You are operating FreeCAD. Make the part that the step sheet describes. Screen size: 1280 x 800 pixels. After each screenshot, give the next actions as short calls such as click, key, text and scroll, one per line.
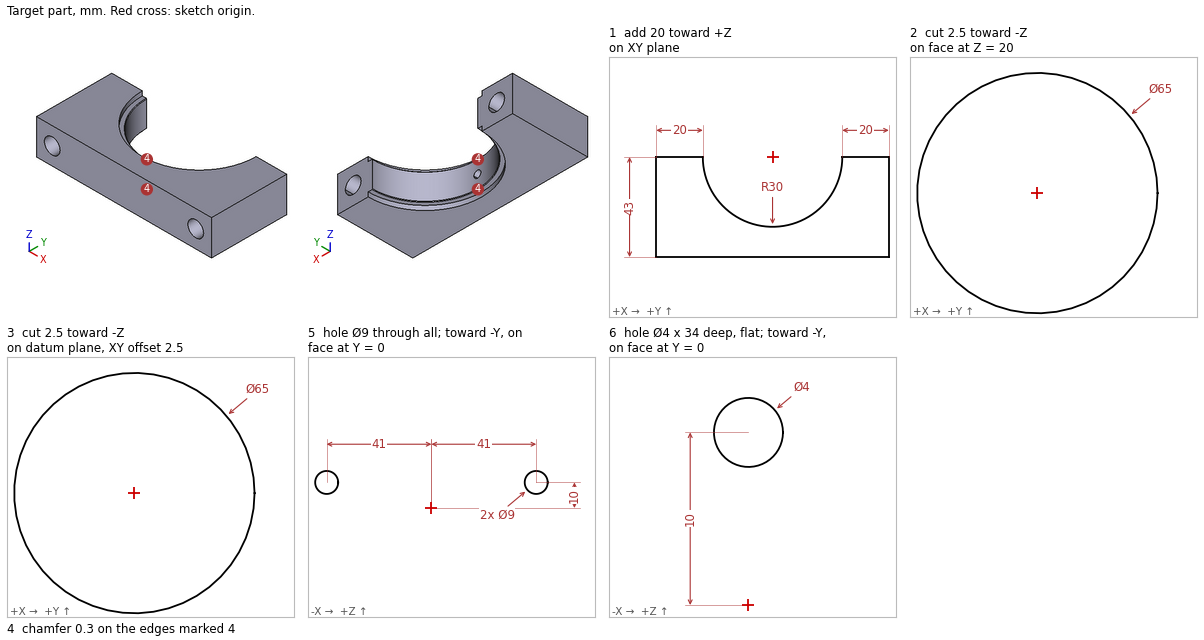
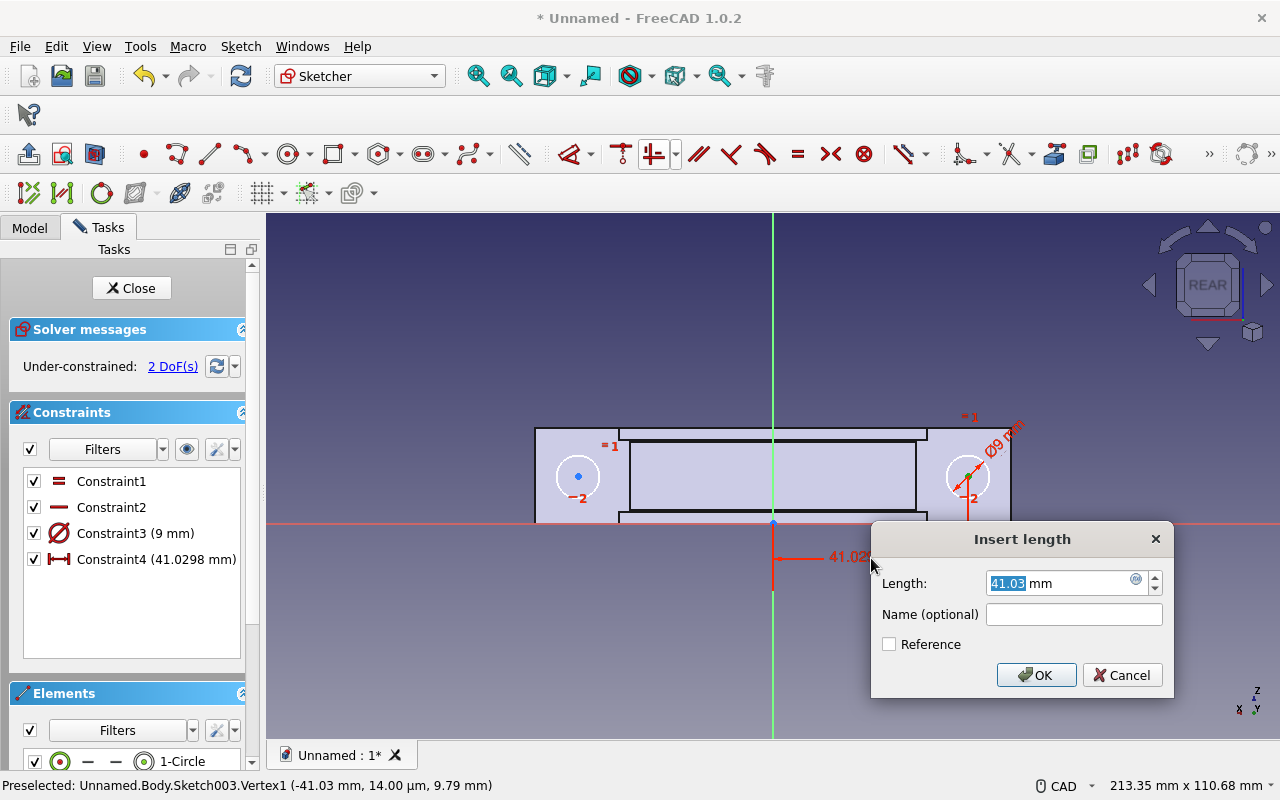
text(41)
key(Return)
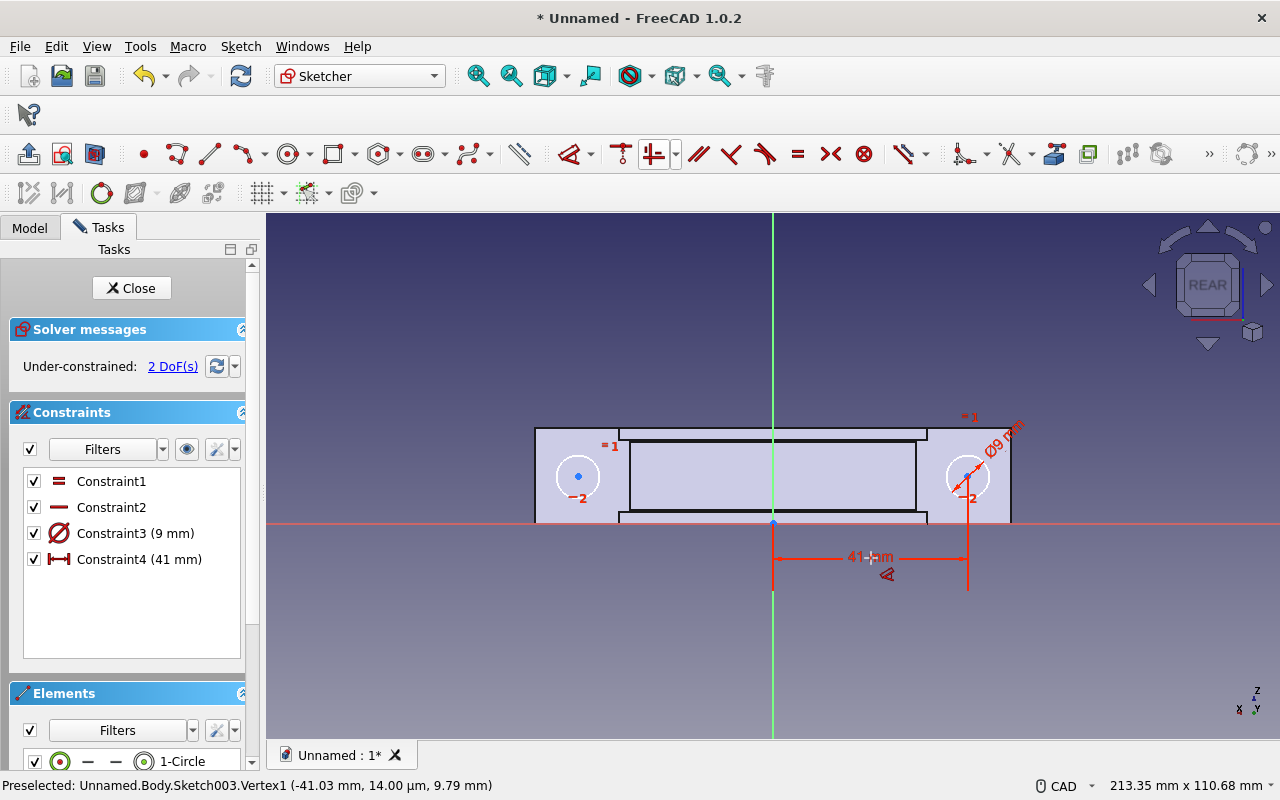
click(968, 477)
click(1002, 500)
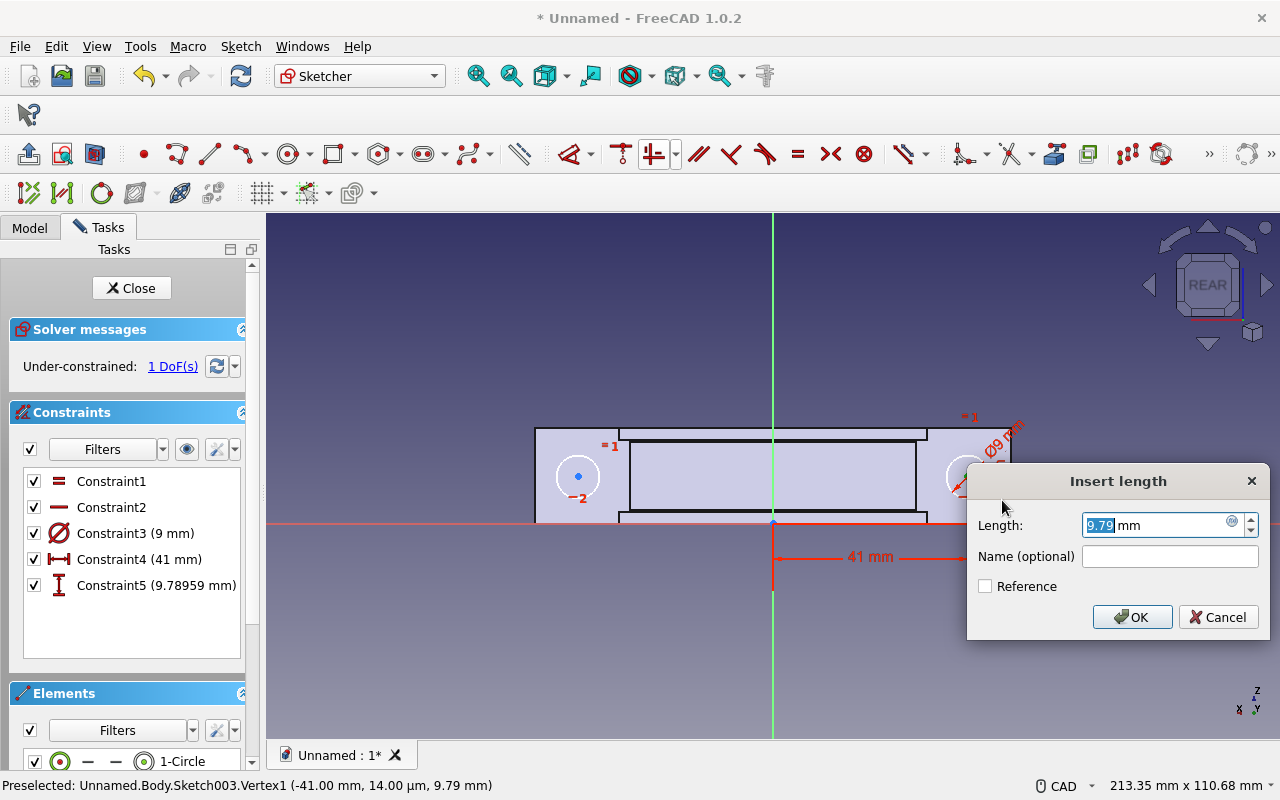
text(10)
key(Return)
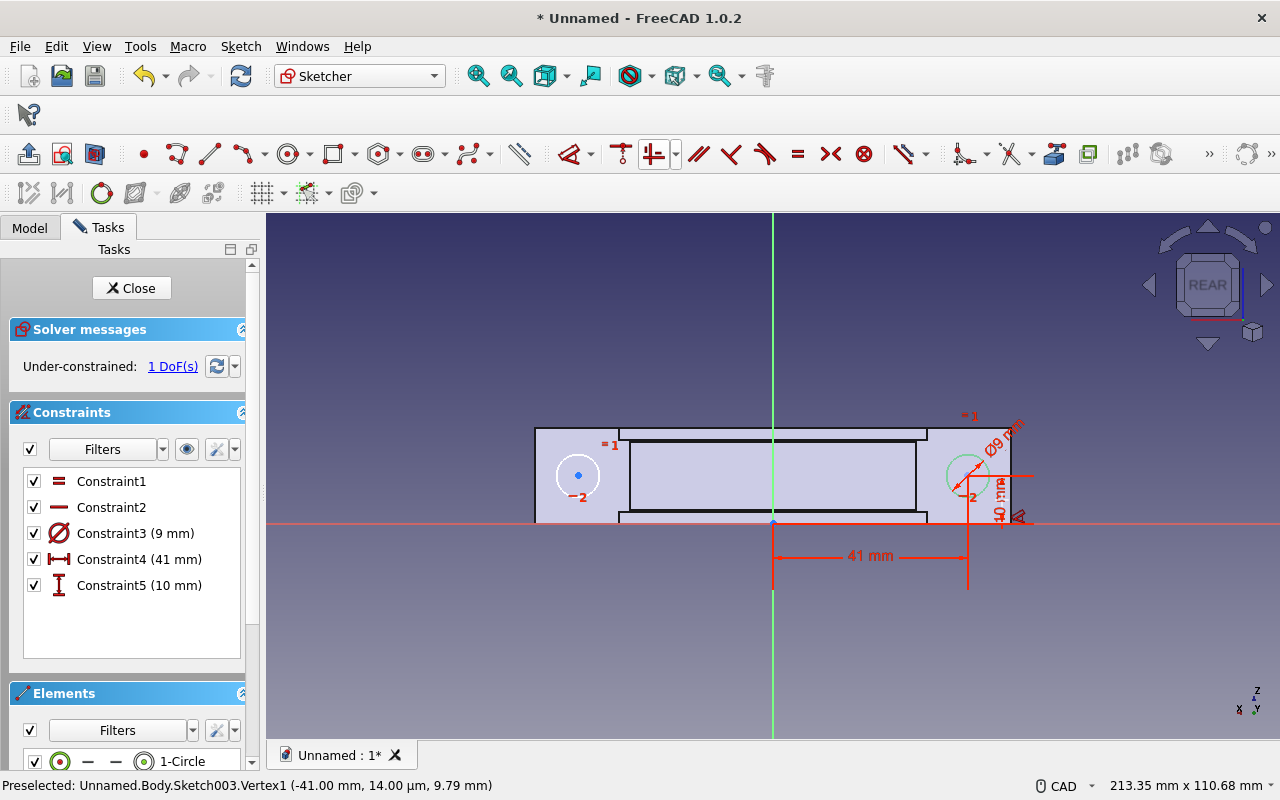
click(578, 476)
click(676, 558)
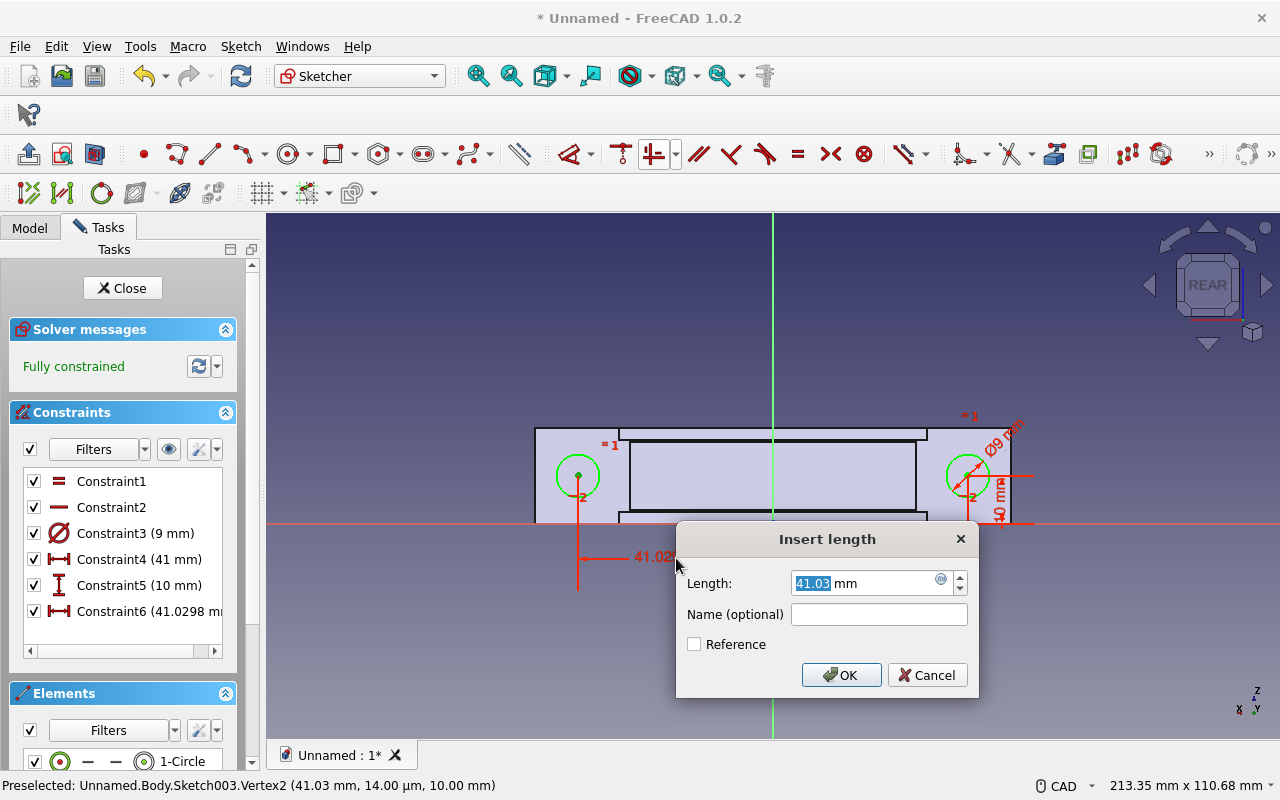
text(41)
key(Return)
key(Escape)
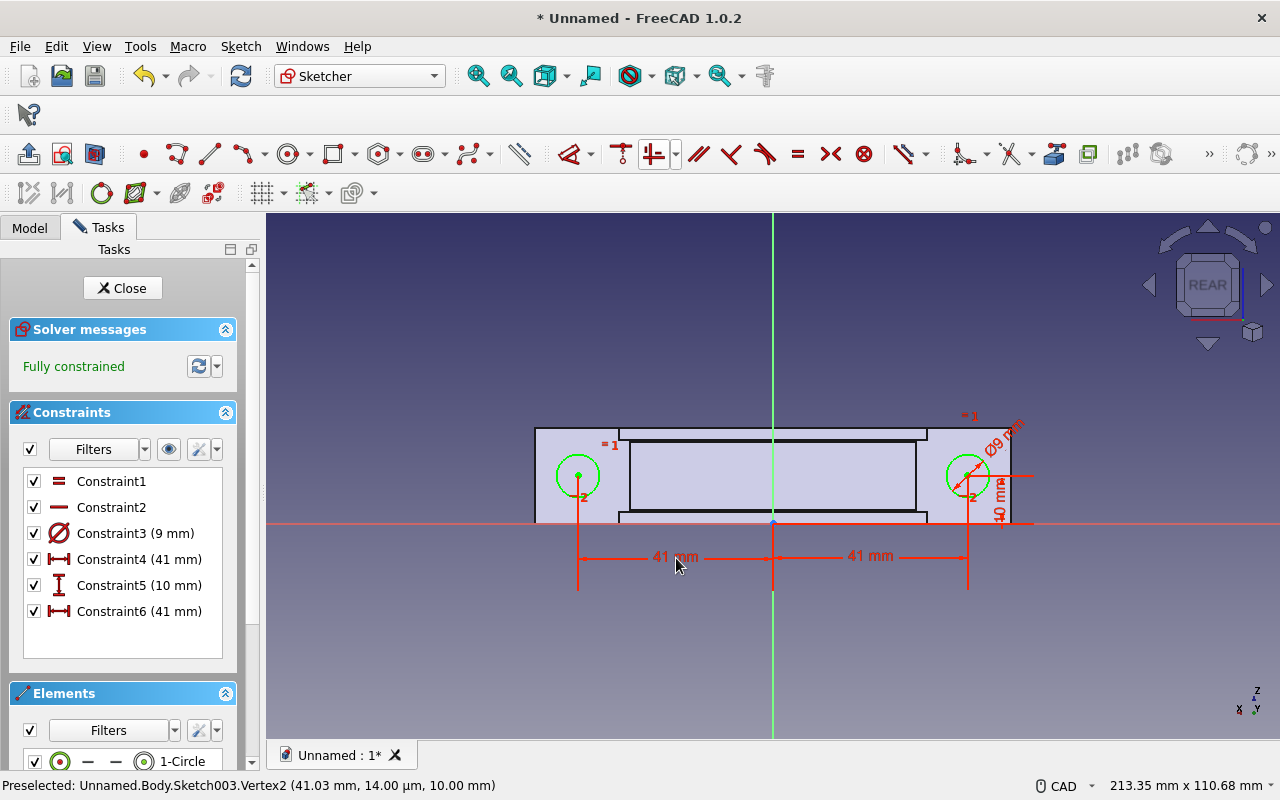
click(123, 288)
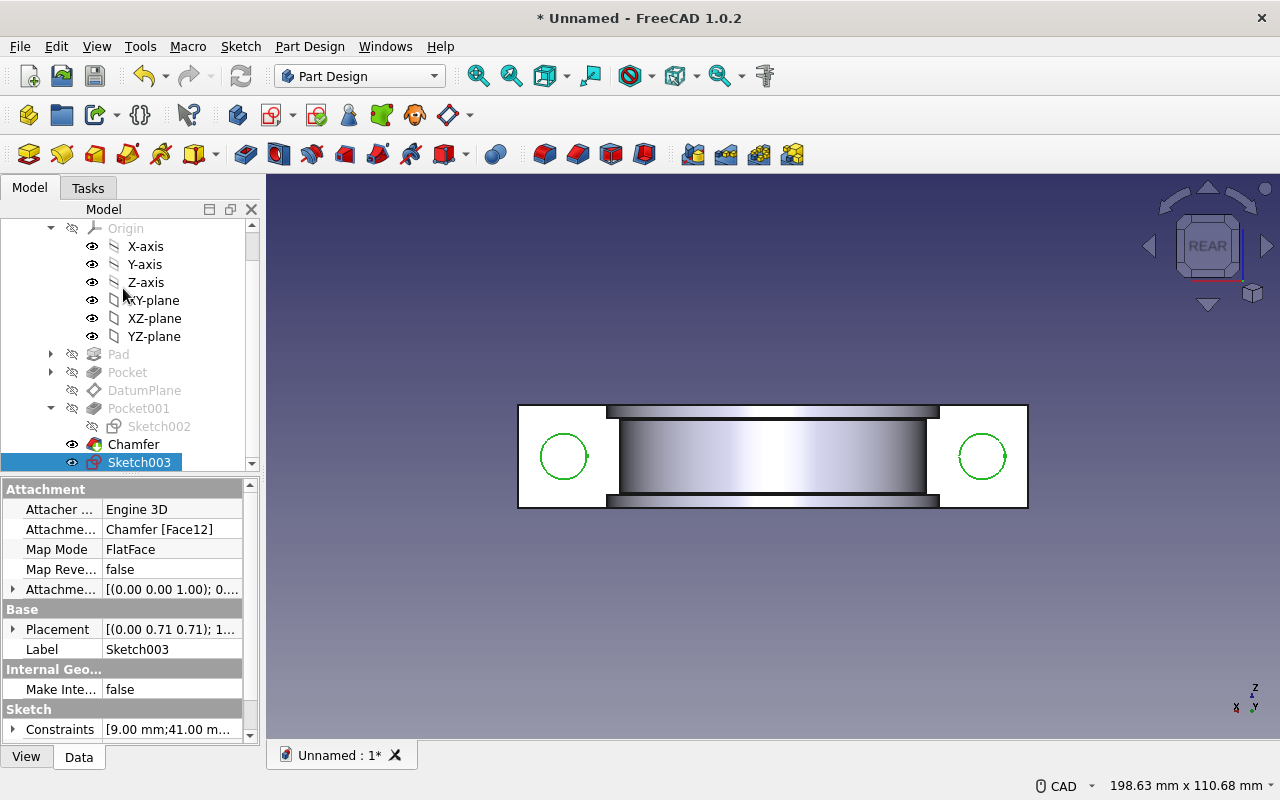
click(279, 154)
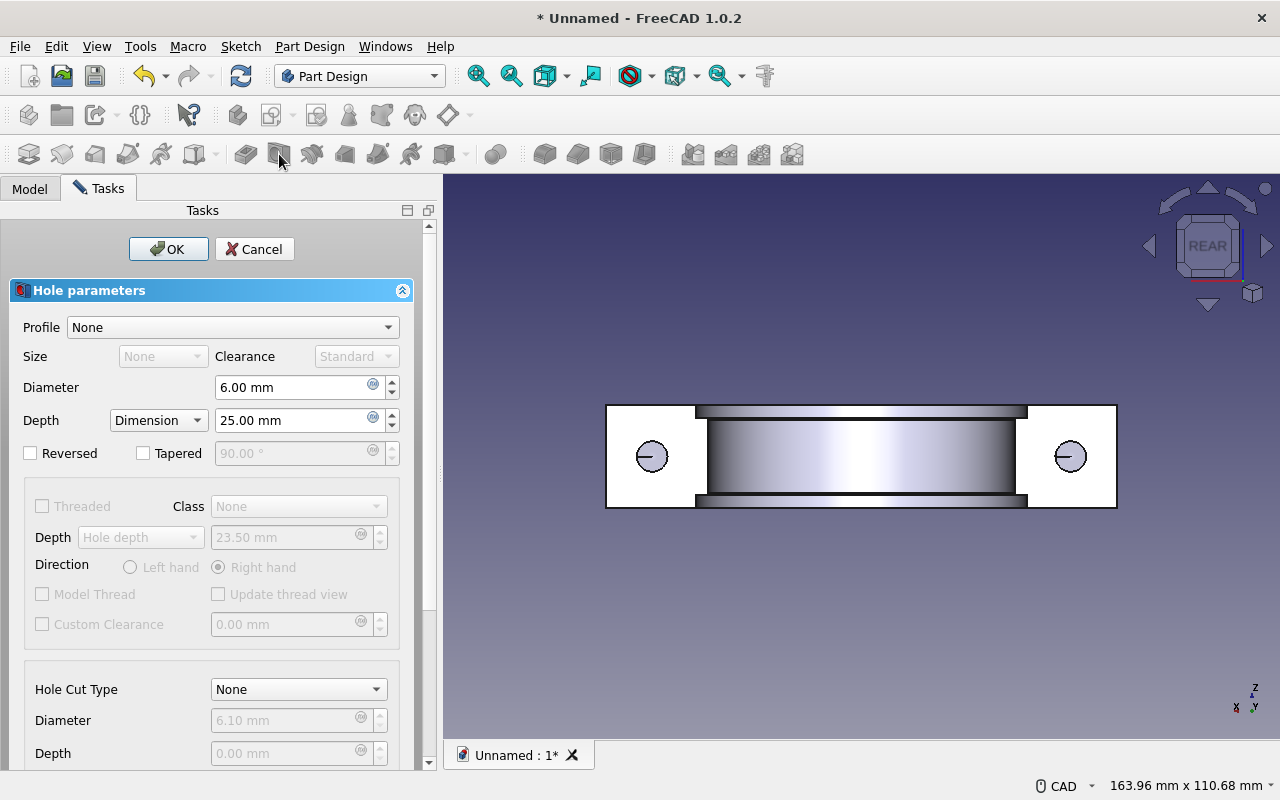
triple_click(300, 388)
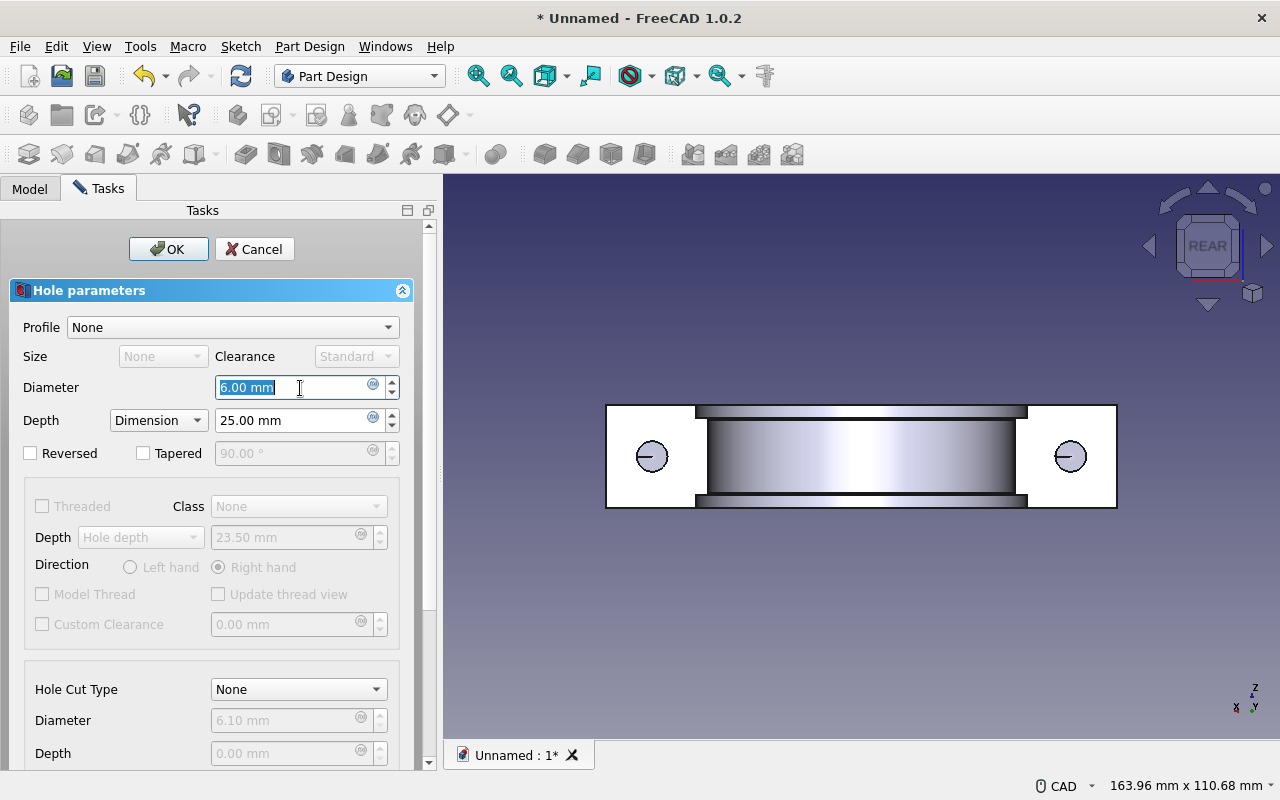
text(9)
key(Tab)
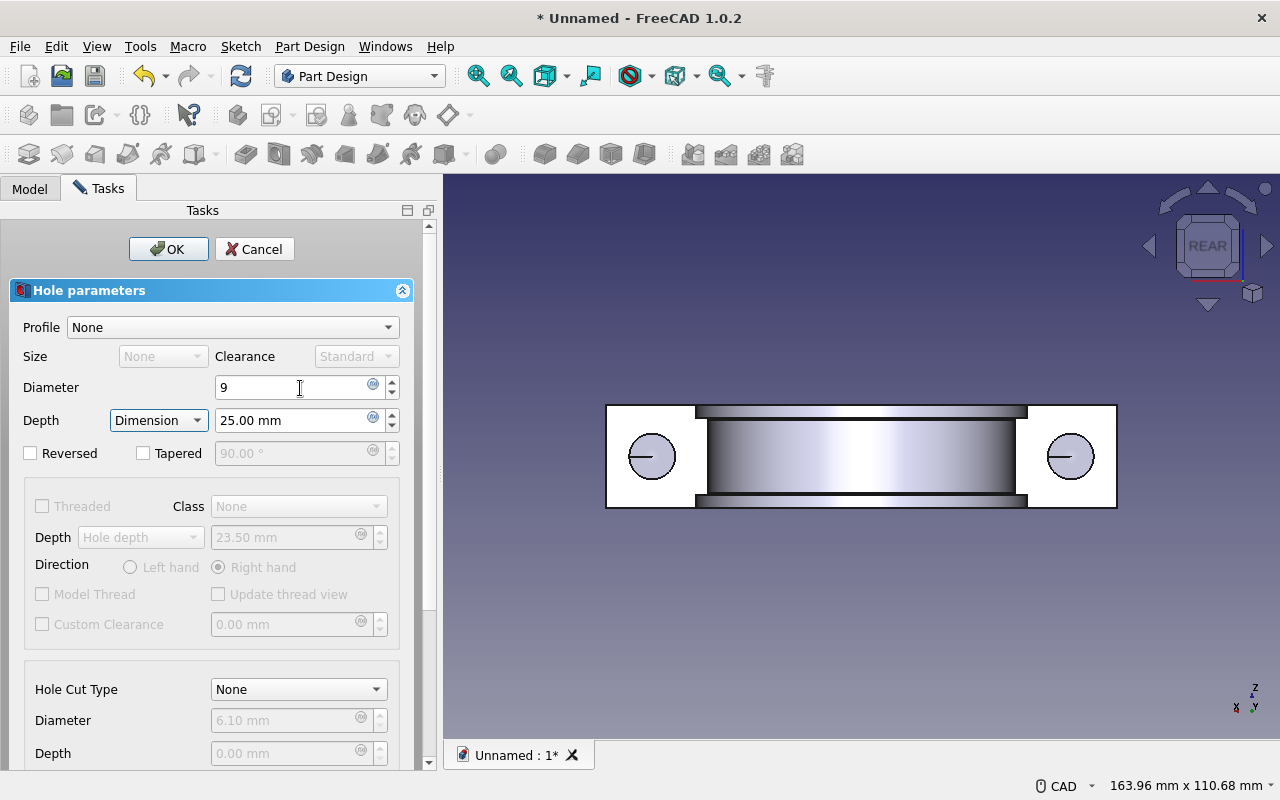
click(160, 420)